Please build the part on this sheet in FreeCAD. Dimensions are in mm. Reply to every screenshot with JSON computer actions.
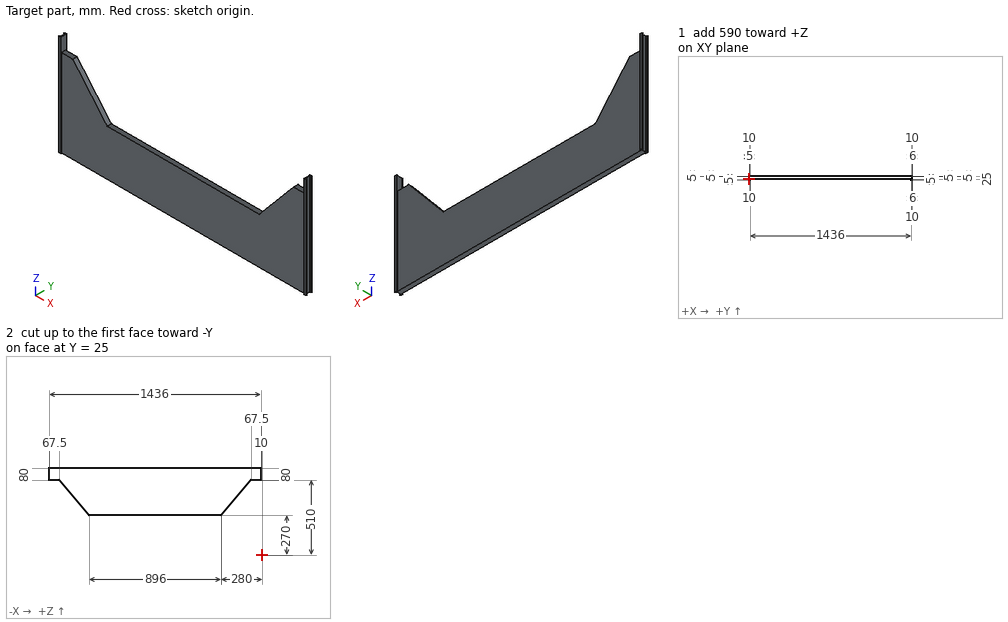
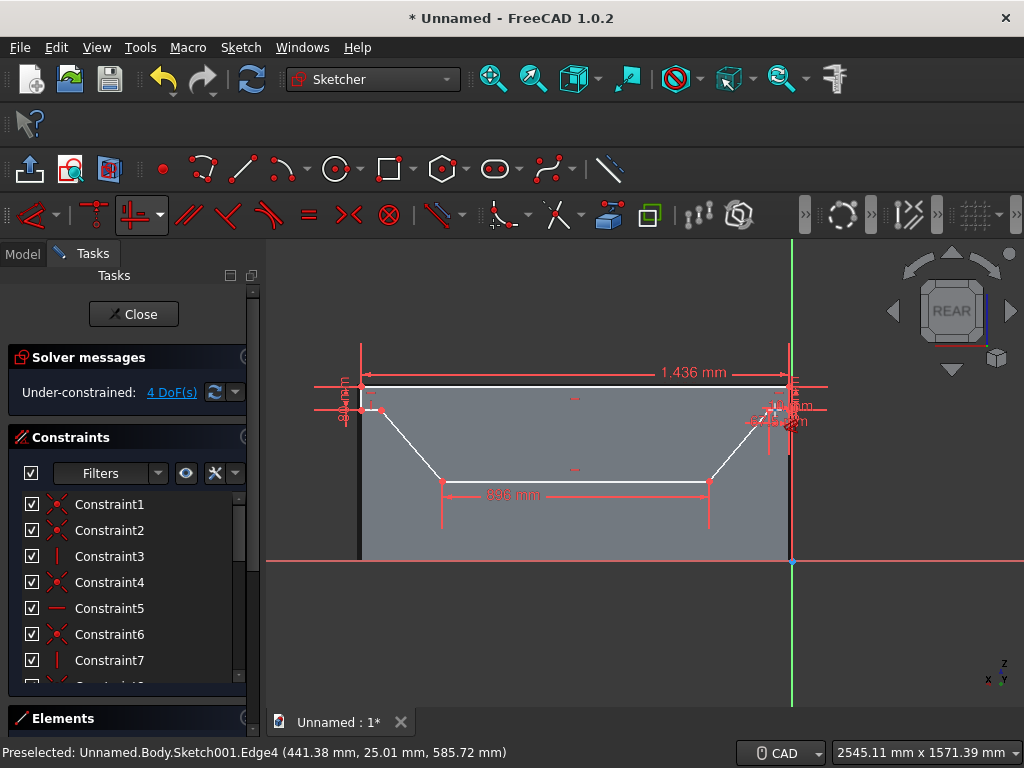
{"action": "scroll", "coordinate": [367, 410], "scroll_direction": "up", "scroll_amount": 5}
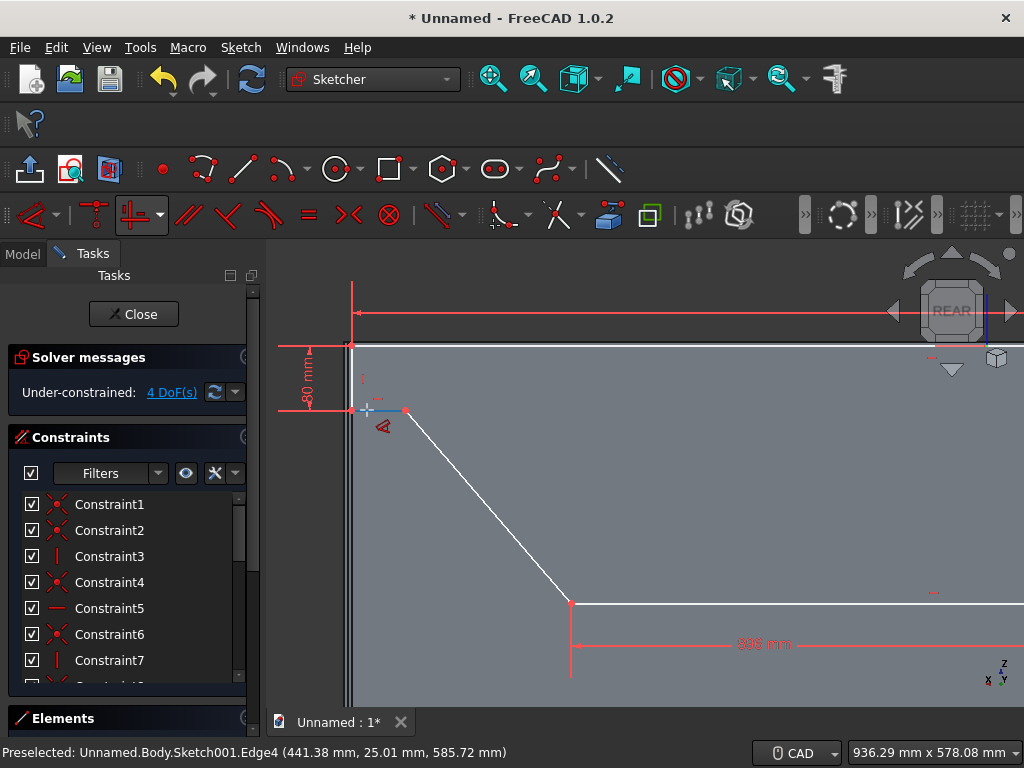
{"action": "left_click", "coordinate": [368, 411]}
{"action": "left_click", "coordinate": [391, 377]}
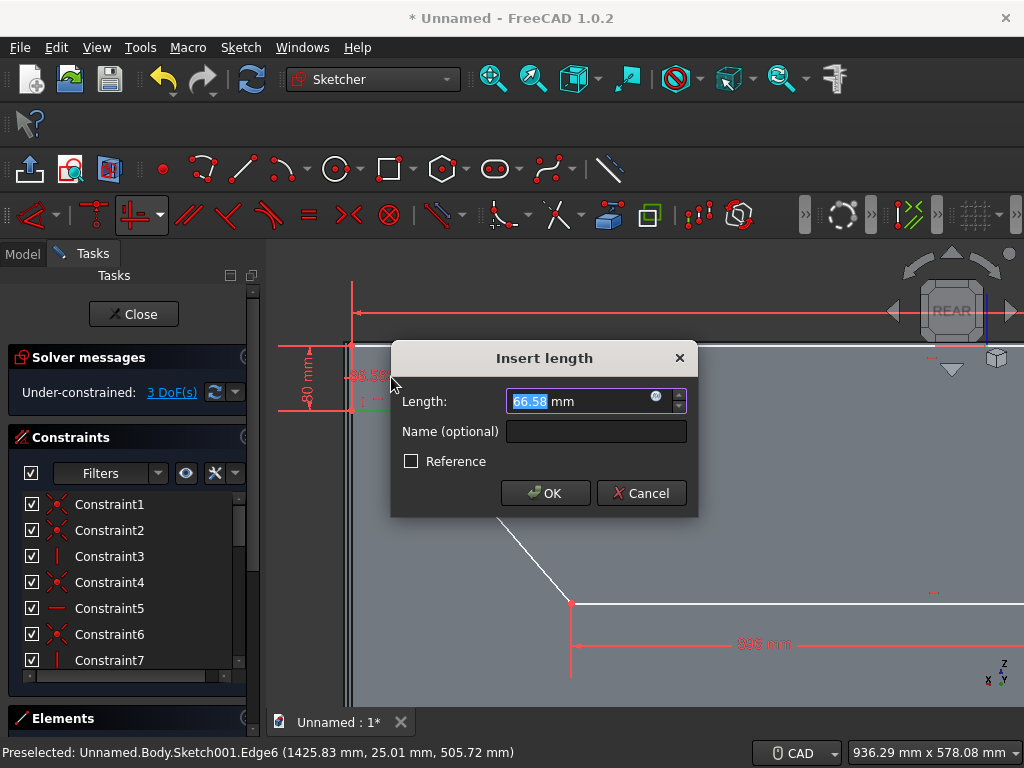
{"action": "type", "text": "67.5"}
{"action": "key", "text": "Return"}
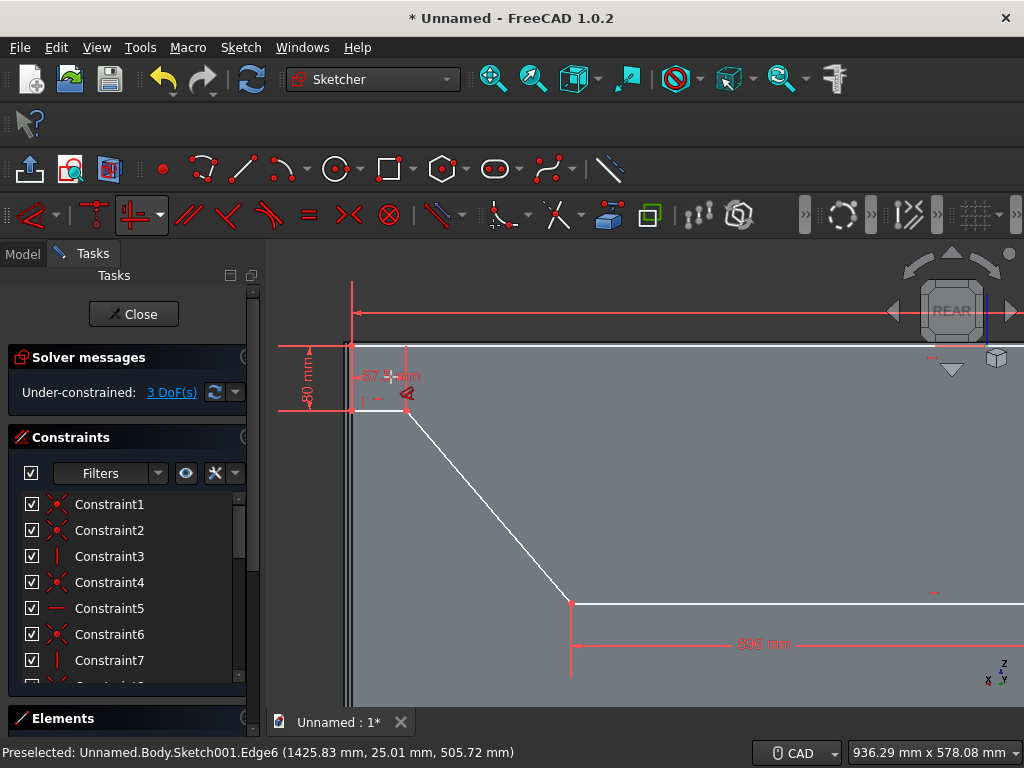
{"action": "scroll", "coordinate": [367, 410], "scroll_direction": "down", "scroll_amount": 5}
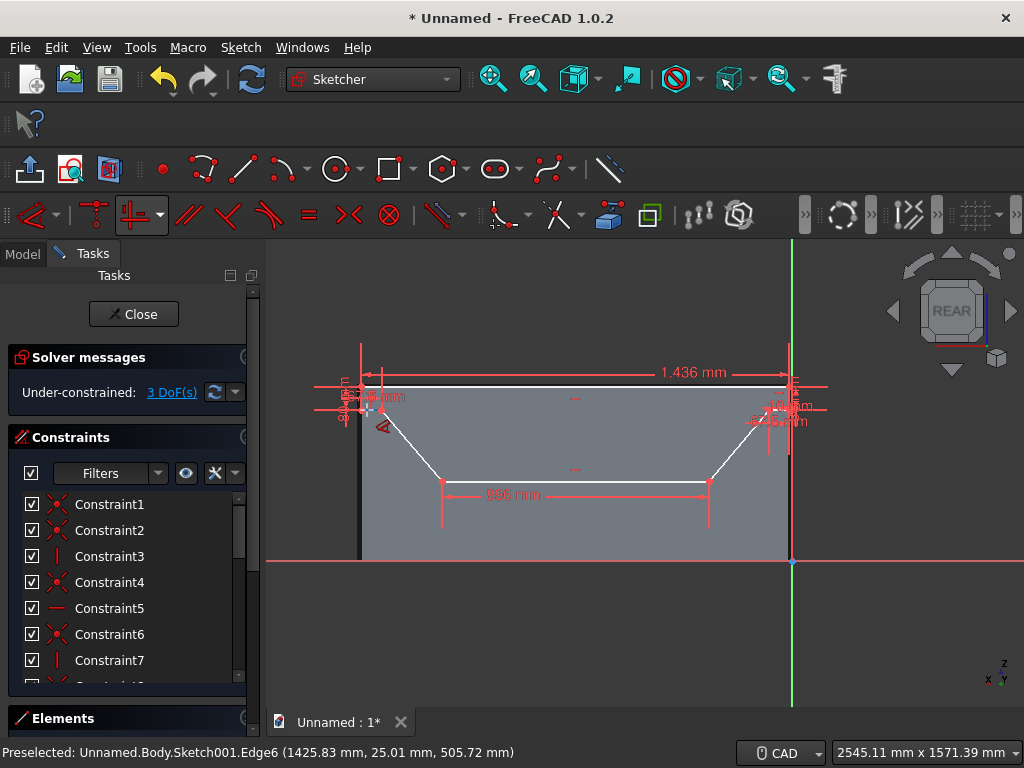
{"action": "left_click", "coordinate": [709, 482]}
{"action": "left_click", "coordinate": [751, 595]}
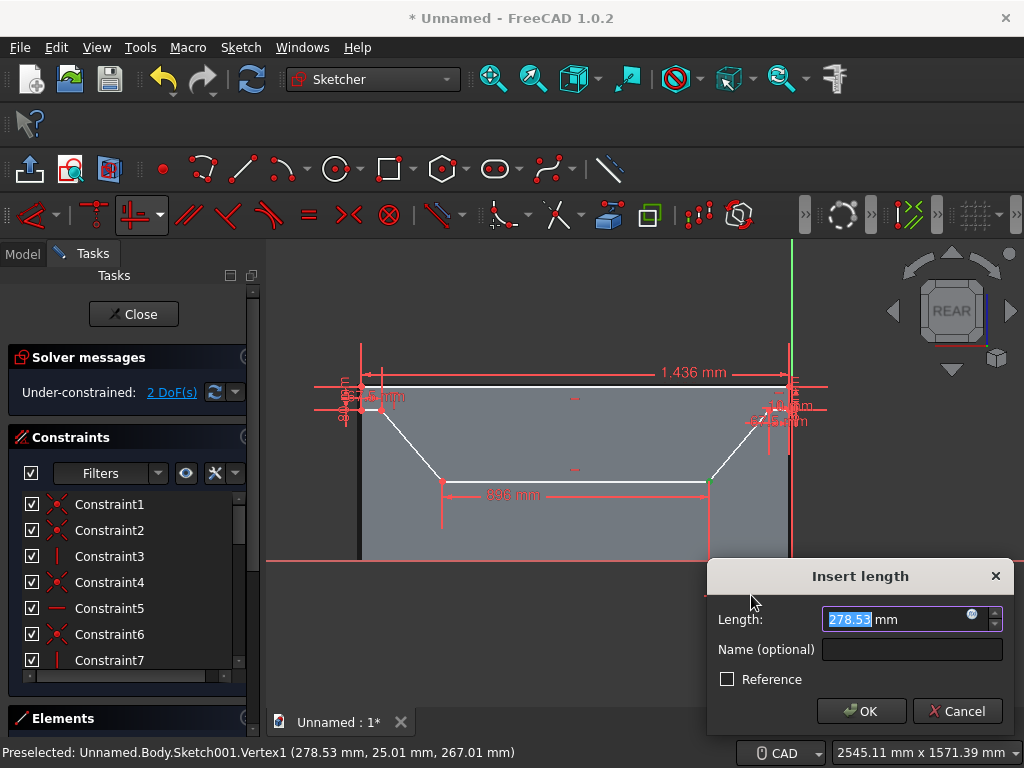
{"action": "type", "text": "280"}
{"action": "key", "text": "Return"}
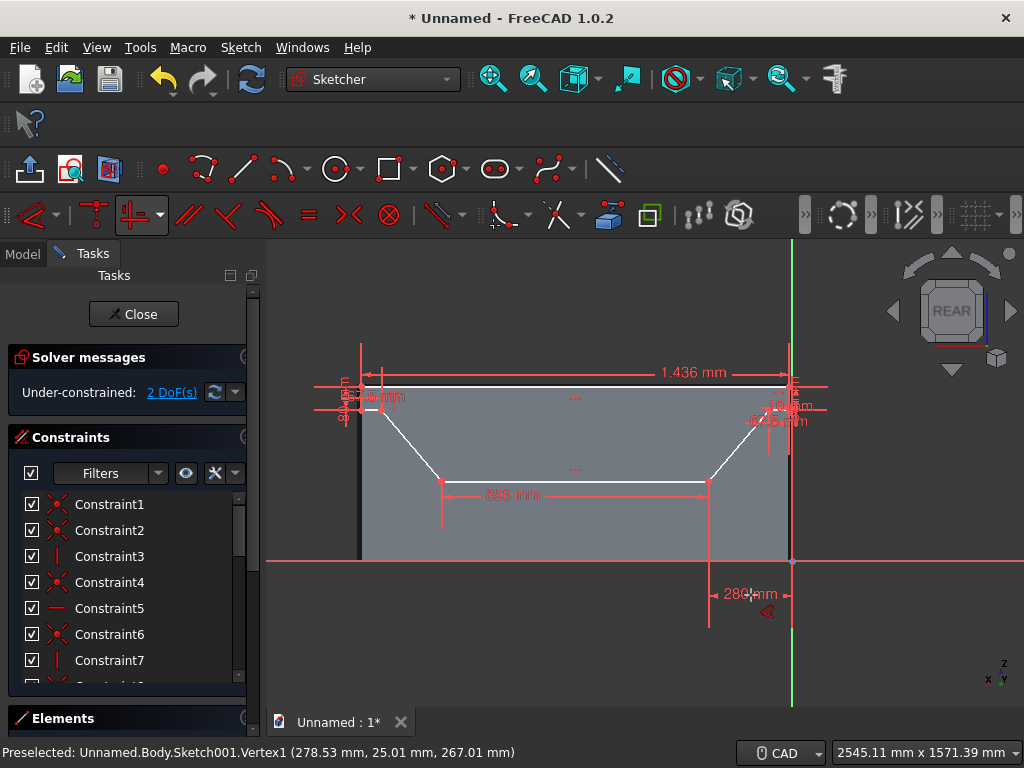
{"action": "left_click", "coordinate": [709, 482]}
{"action": "left_click", "coordinate": [826, 521]}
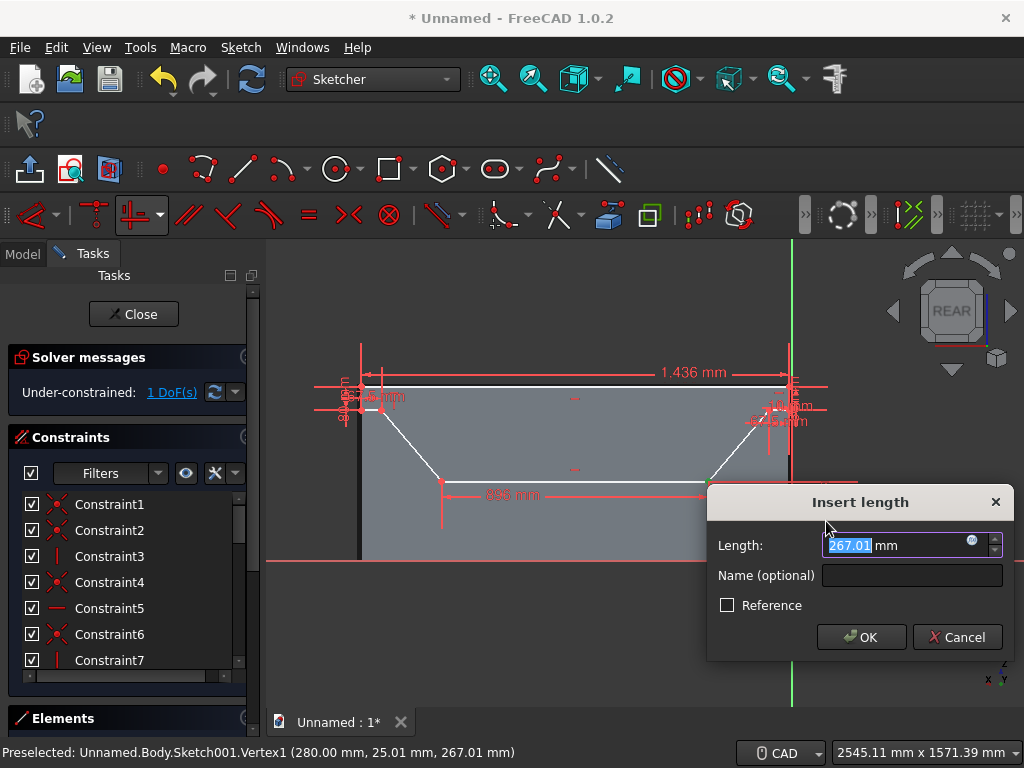
{"action": "type", "text": "270"}
{"action": "key", "text": "Return"}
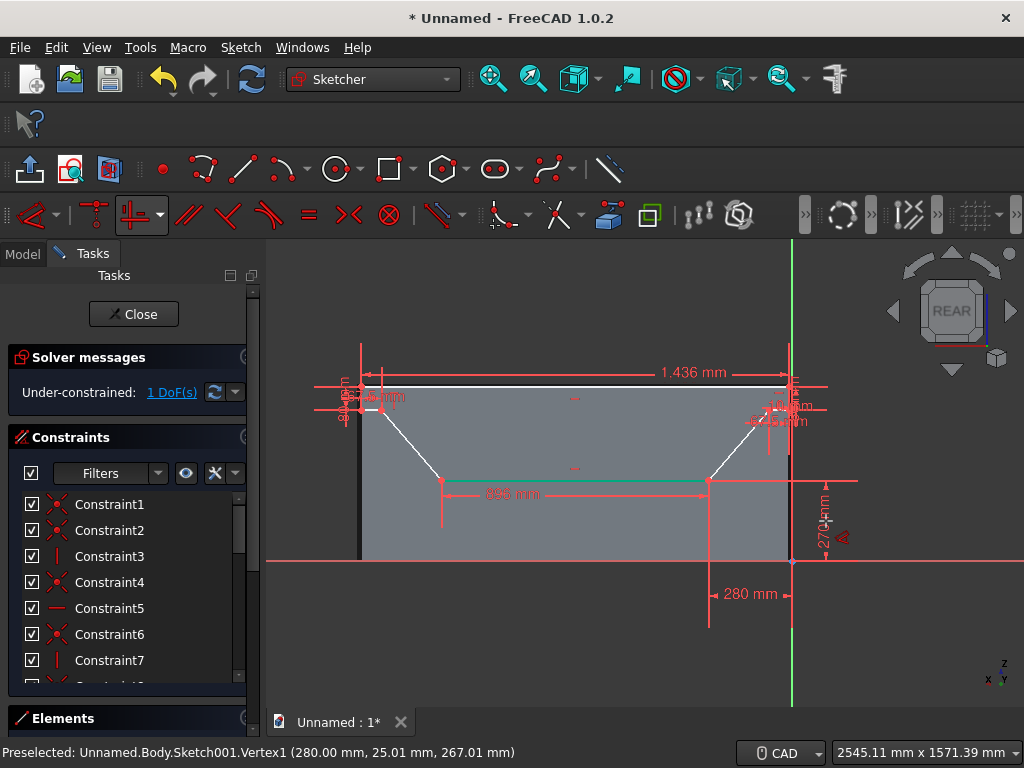
{"action": "left_click", "coordinate": [769, 410]}
{"action": "left_click", "coordinate": [826, 486]}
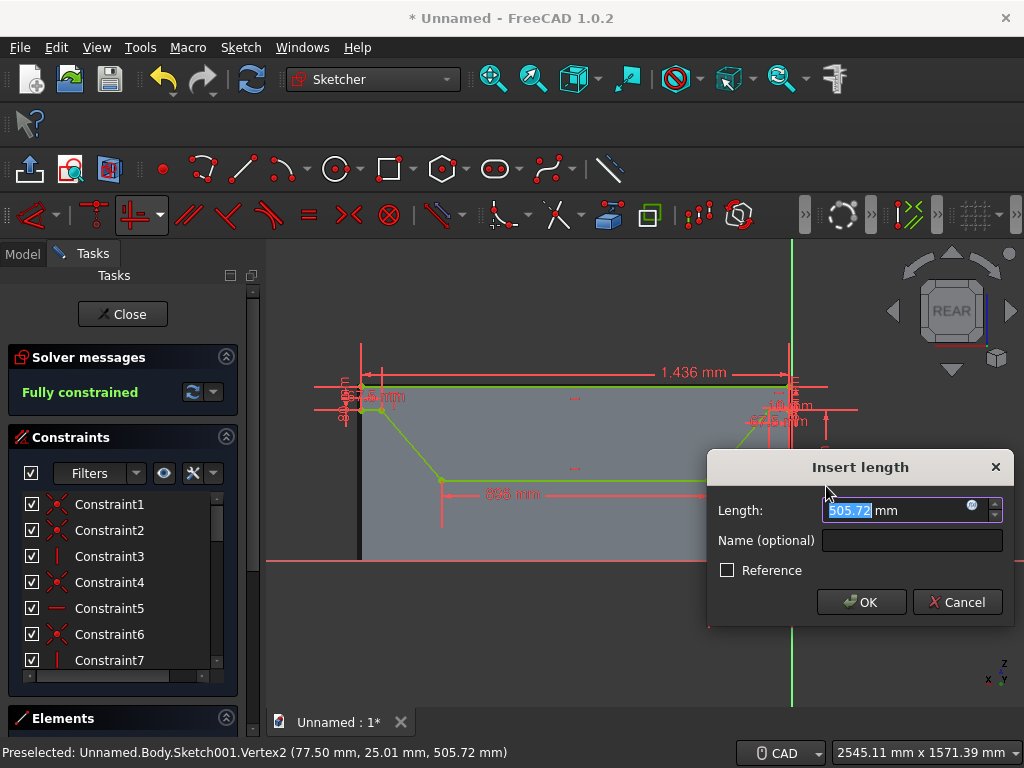
{"action": "type", "text": "510"}
{"action": "key", "text": "Return"}
{"action": "key", "text": "Escape"}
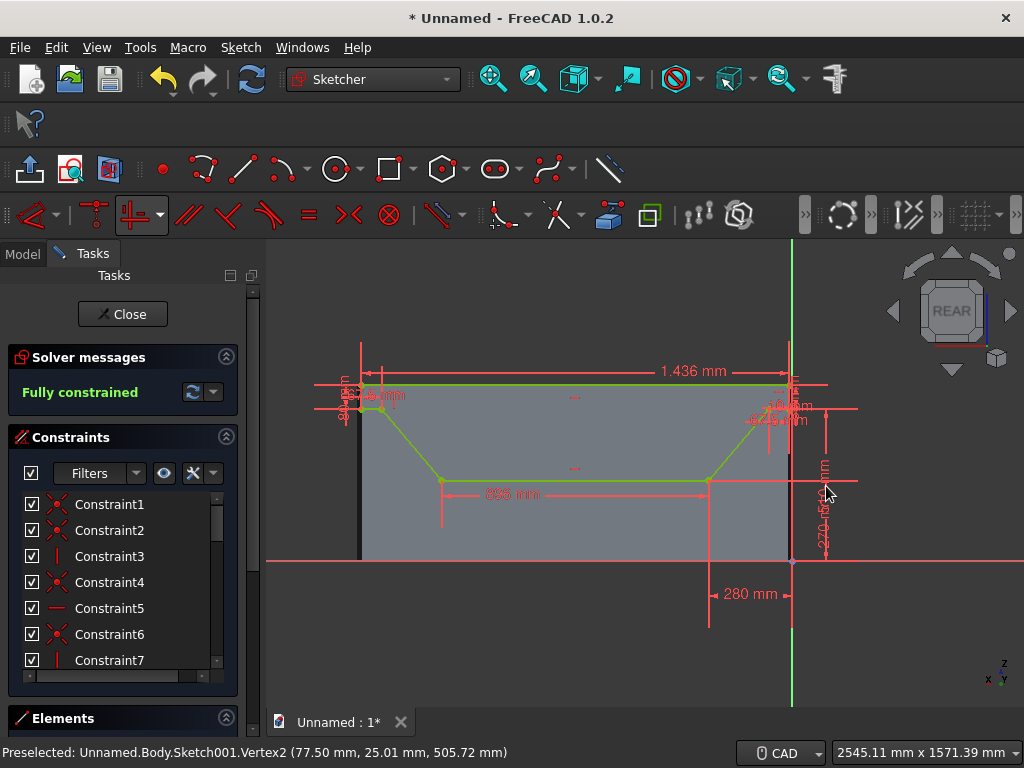
{"action": "left_click", "coordinate": [123, 314]}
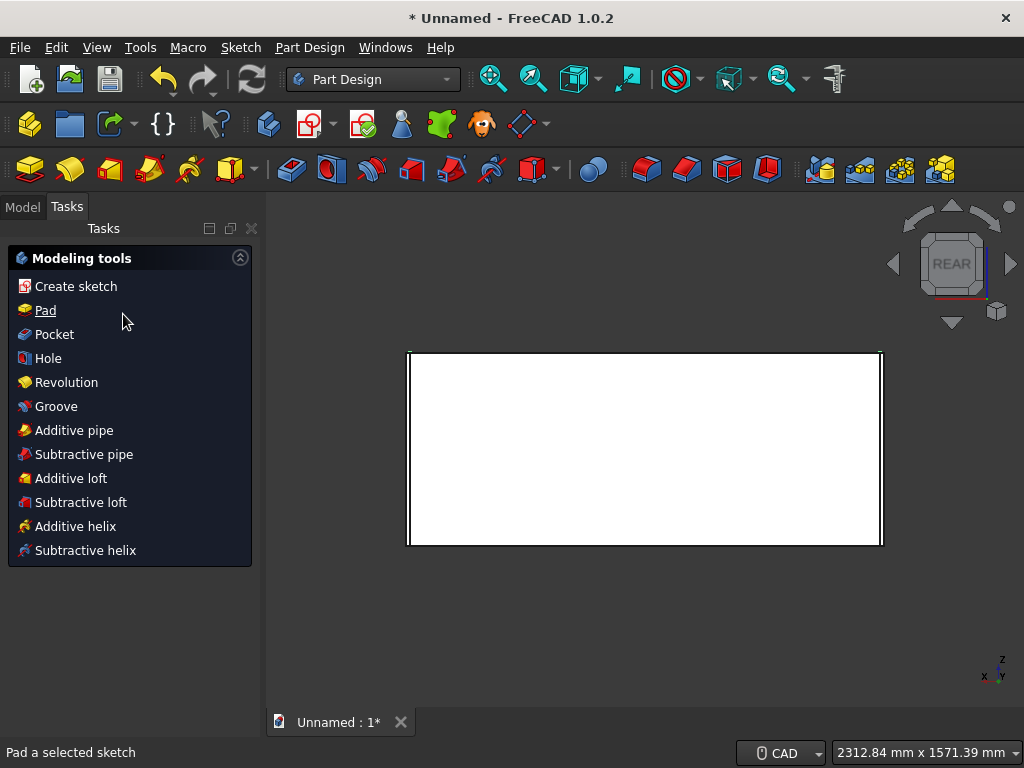
{"action": "left_click", "coordinate": [292, 170]}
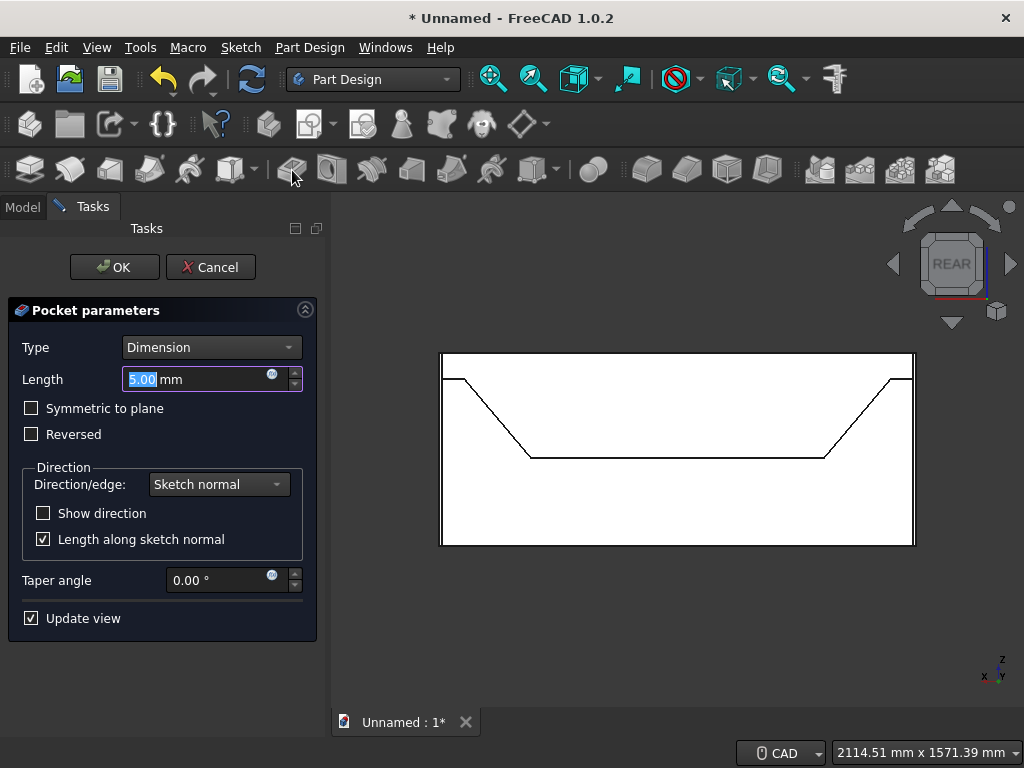
{"action": "left_click", "coordinate": [212, 348]}